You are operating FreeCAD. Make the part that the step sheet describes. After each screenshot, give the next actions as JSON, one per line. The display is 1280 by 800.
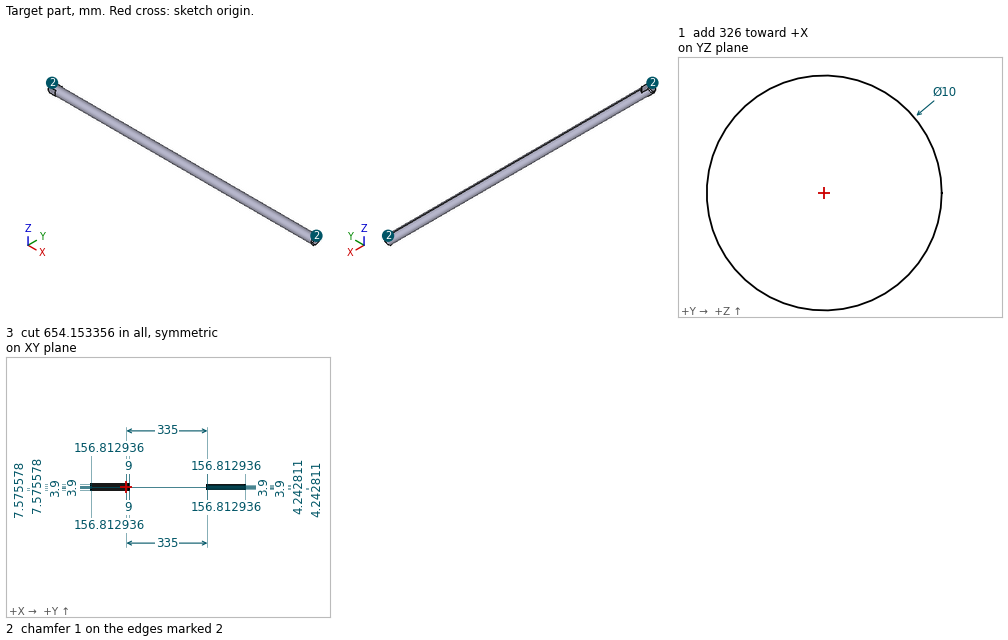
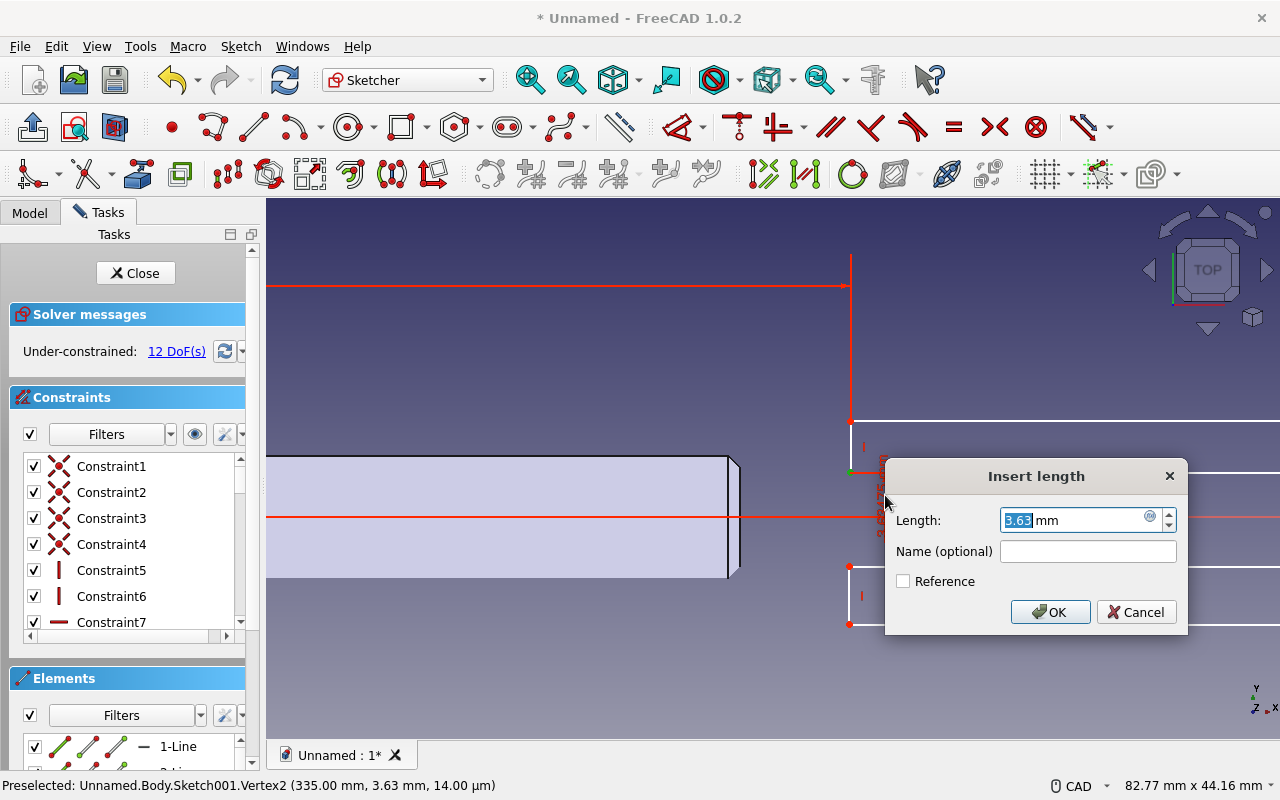
{"action": "type", "text": "3.9"}
{"action": "key", "text": "Return"}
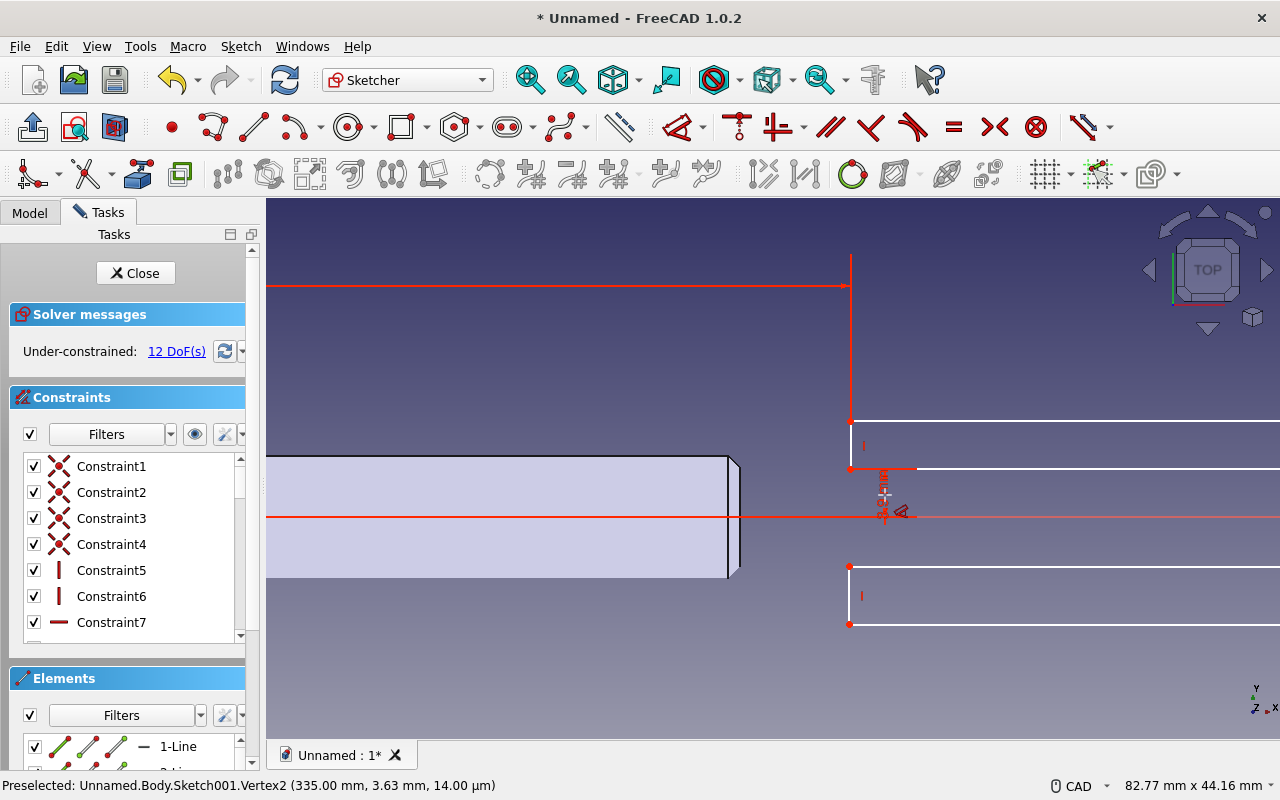
{"action": "scroll", "coordinate": [853, 465], "scroll_direction": "down", "scroll_amount": 13}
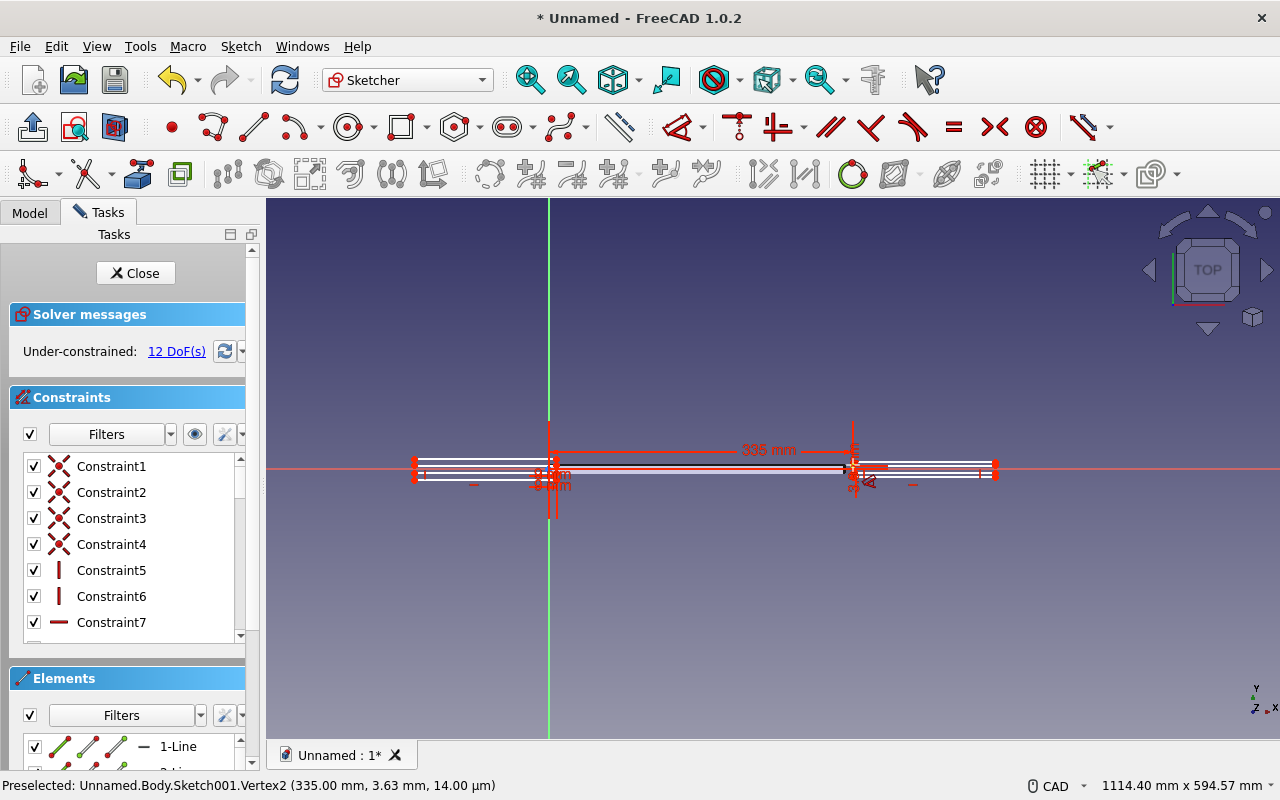
{"action": "scroll", "coordinate": [853, 473], "scroll_direction": "up", "scroll_amount": 6}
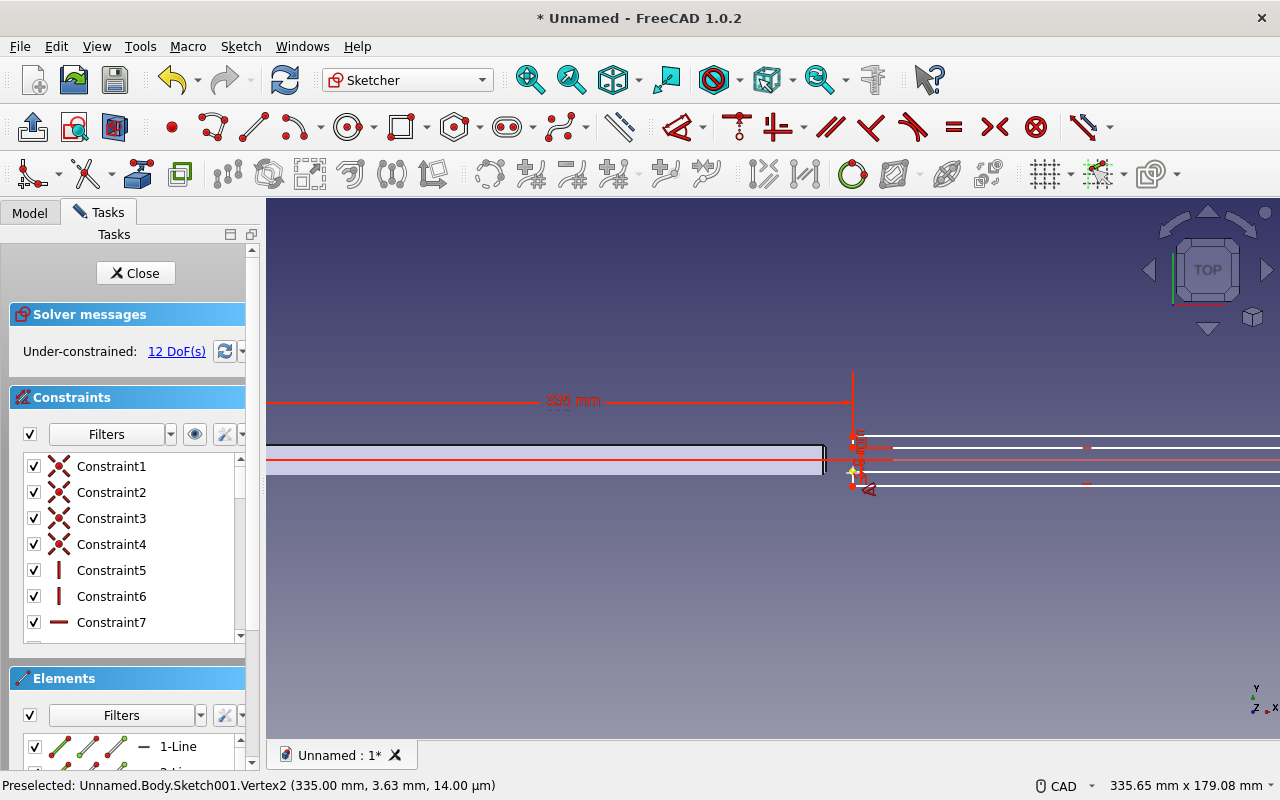
{"action": "left_click", "coordinate": [853, 472]}
{"action": "left_click", "coordinate": [573, 506]}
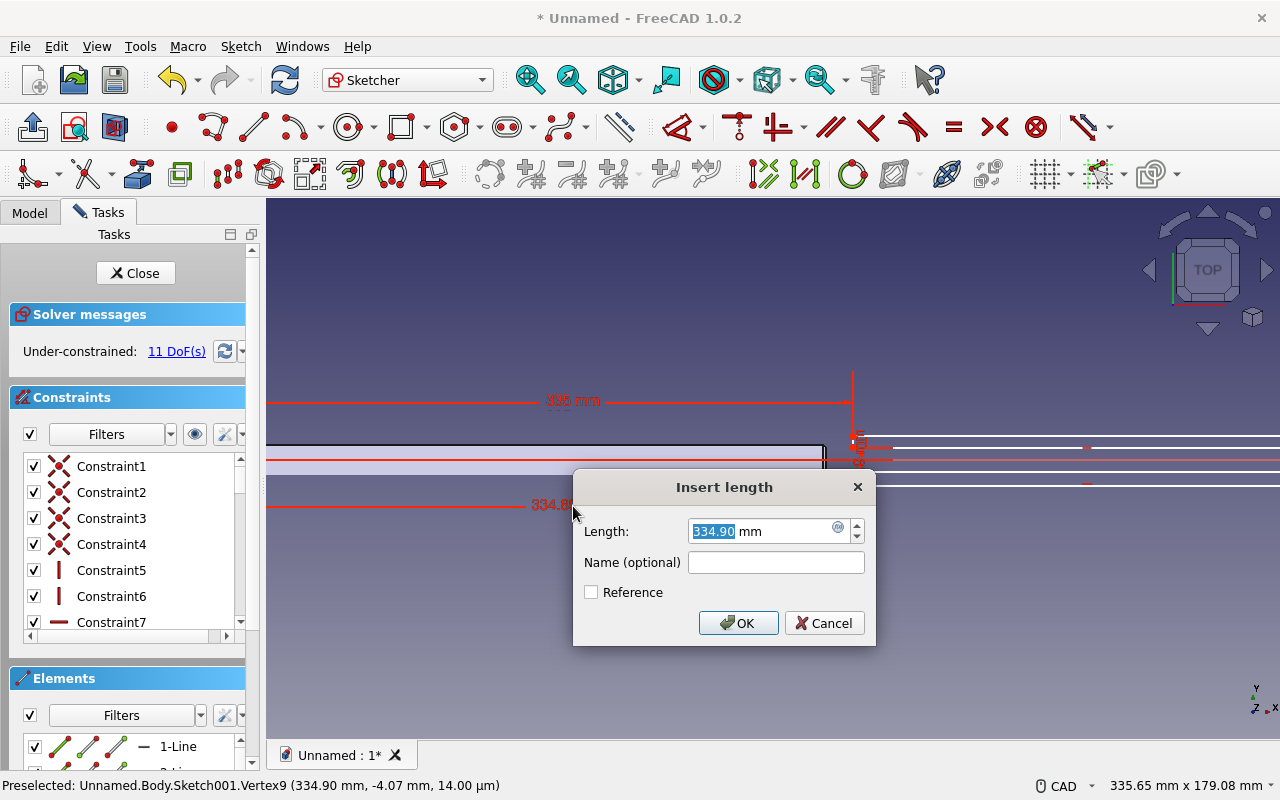
{"action": "type", "text": "335"}
{"action": "key", "text": "Return"}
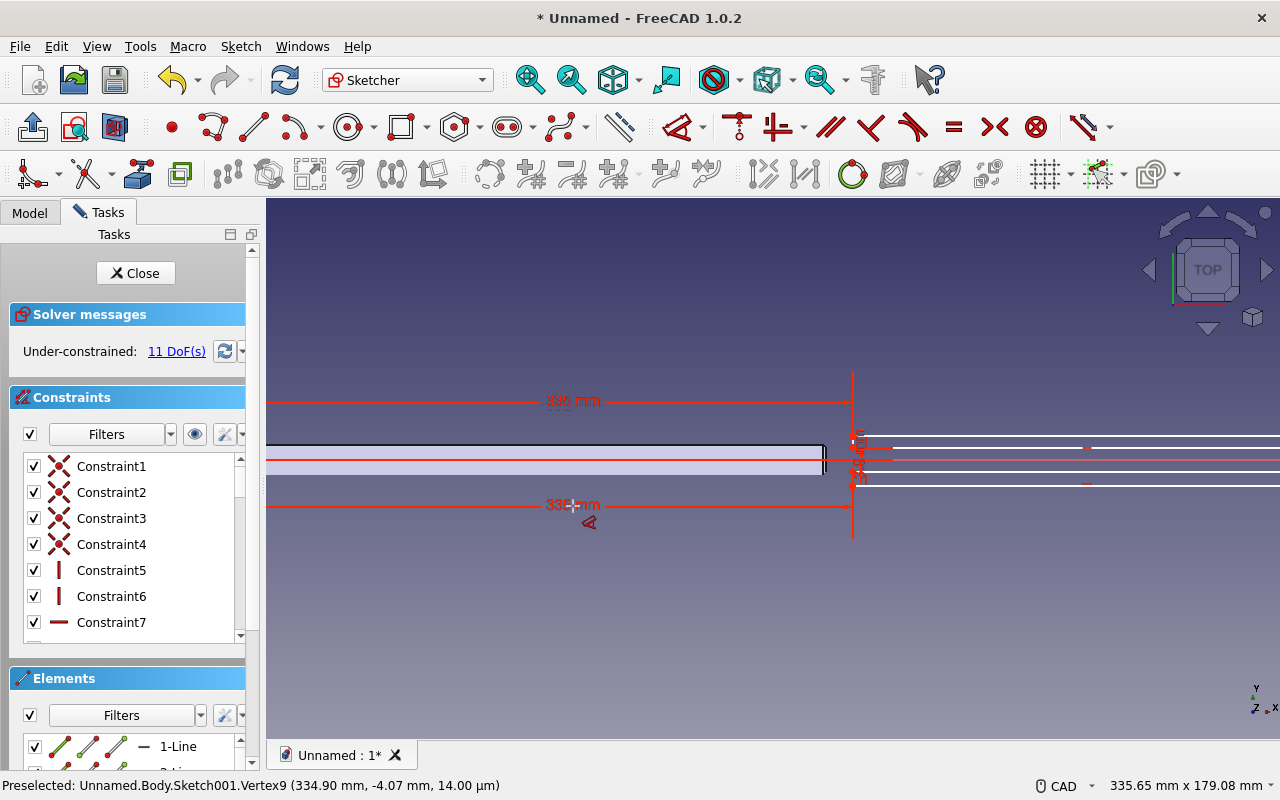
{"action": "scroll", "coordinate": [853, 472], "scroll_direction": "up", "scroll_amount": 7}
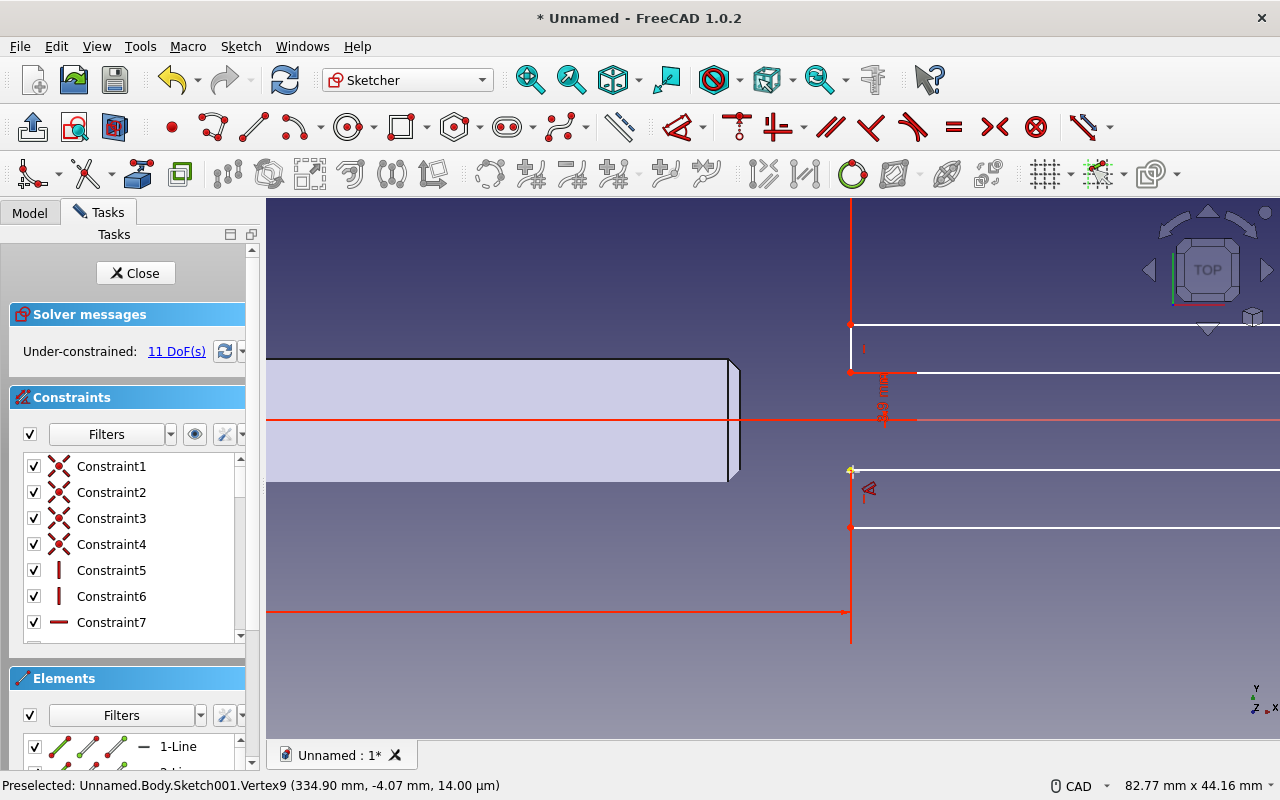
{"action": "left_click", "coordinate": [851, 470]}
{"action": "left_click", "coordinate": [885, 445]}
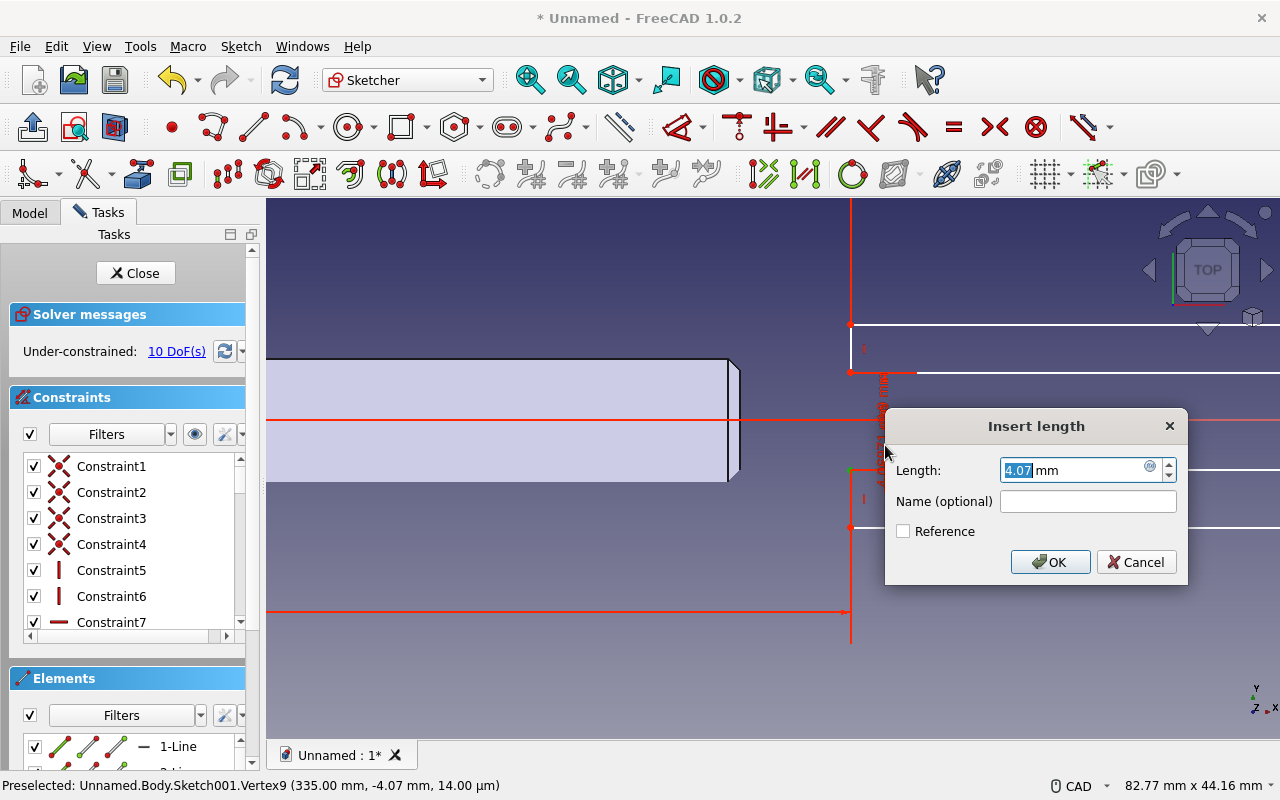
{"action": "type", "text": "3.9"}
{"action": "key", "text": "Return"}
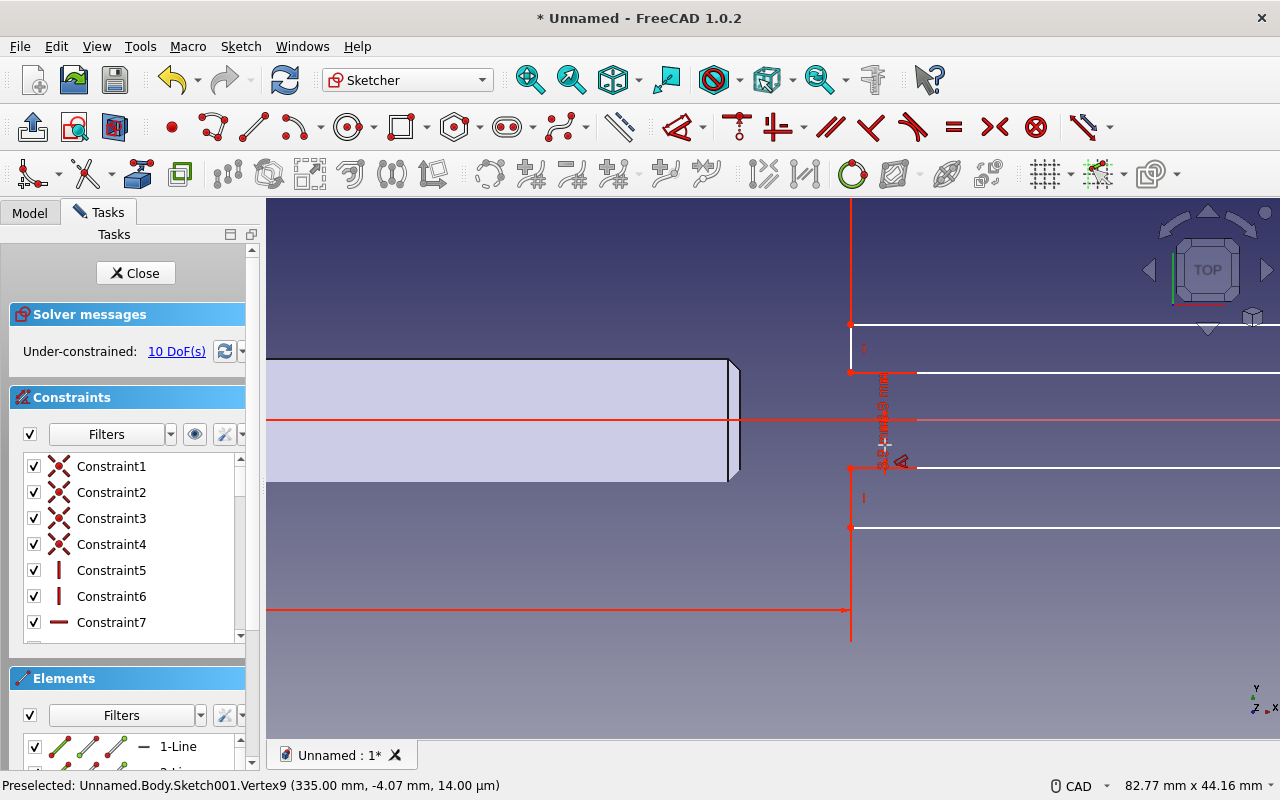
{"action": "scroll", "coordinate": [853, 472], "scroll_direction": "down", "scroll_amount": 13}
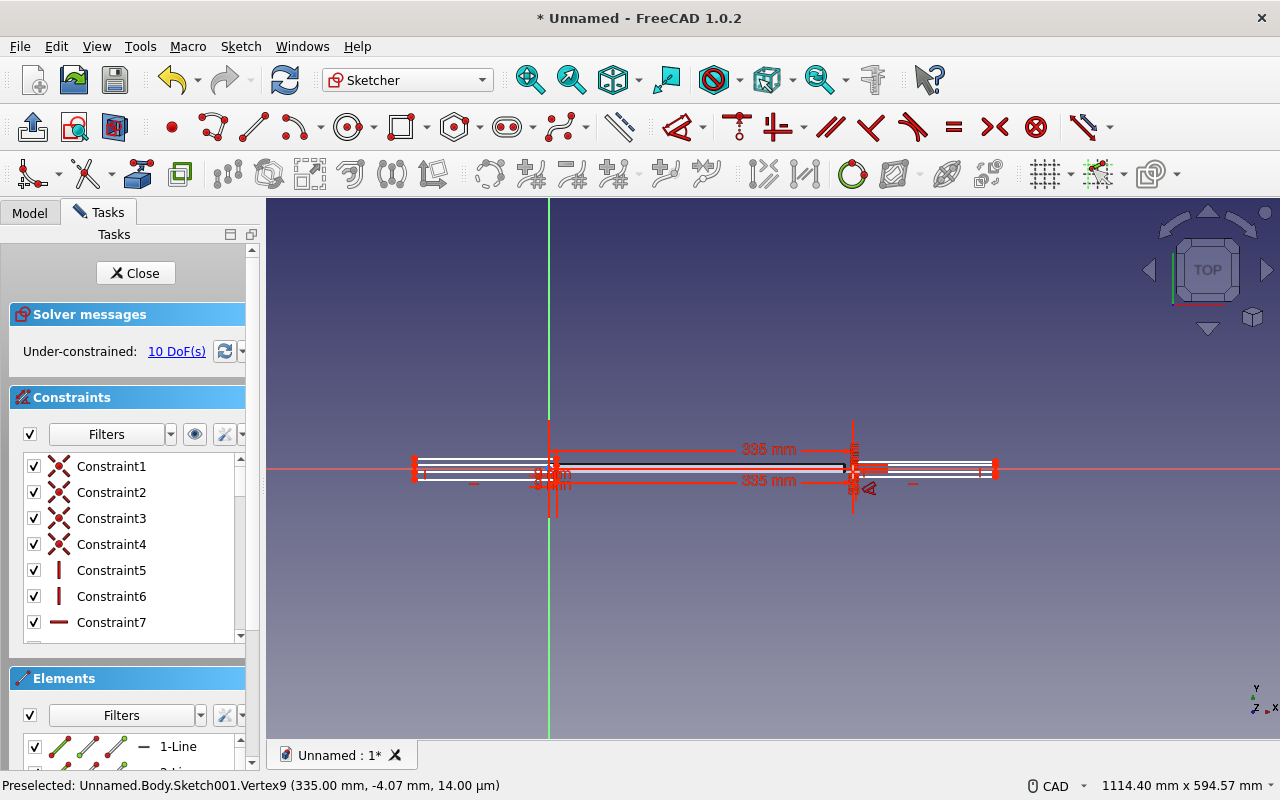
{"action": "scroll", "coordinate": [414, 465], "scroll_direction": "up", "scroll_amount": 13}